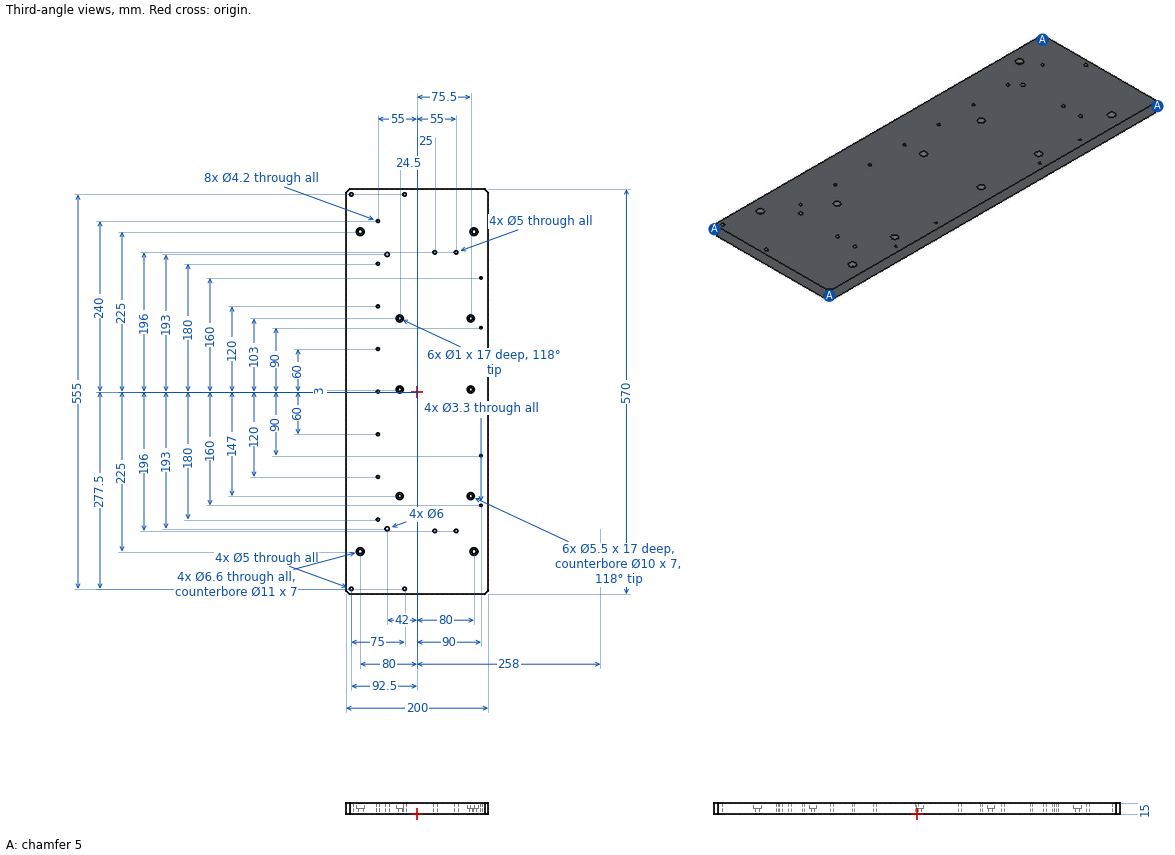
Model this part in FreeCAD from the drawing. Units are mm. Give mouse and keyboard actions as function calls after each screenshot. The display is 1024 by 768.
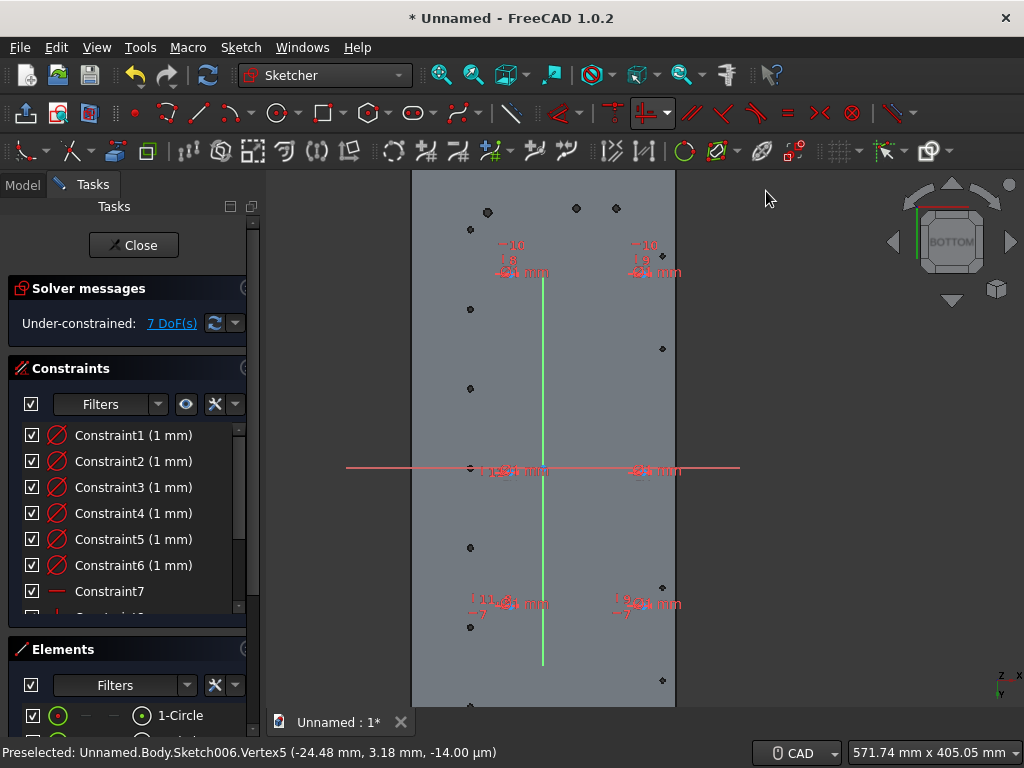
click(643, 606)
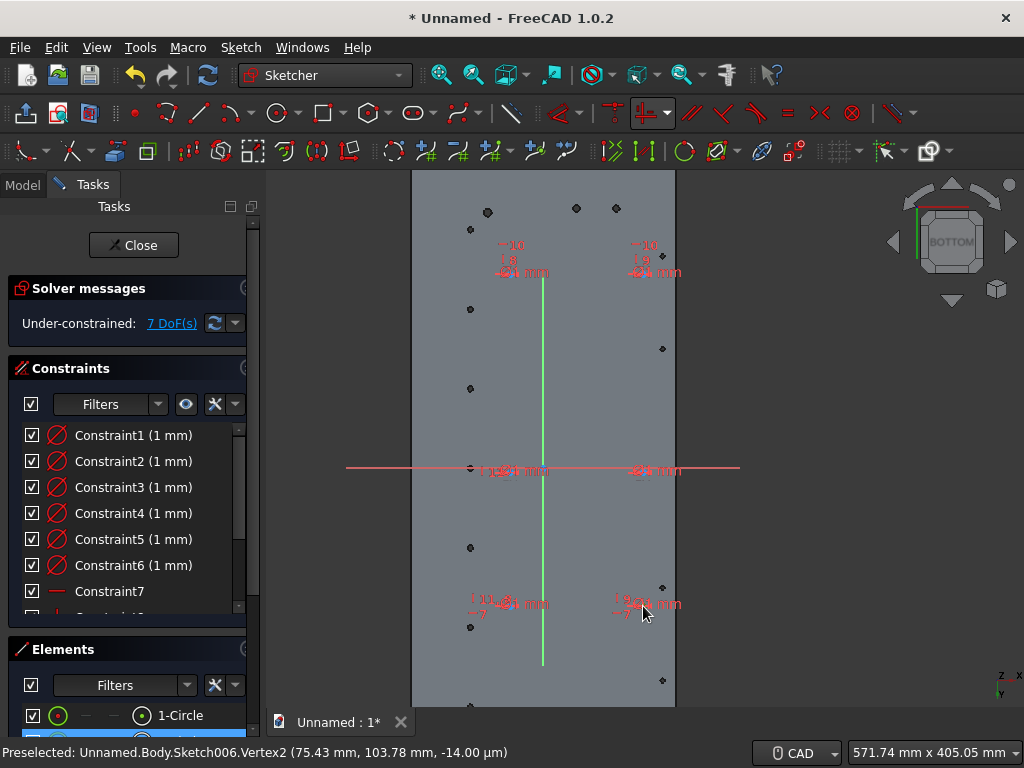
click(643, 473)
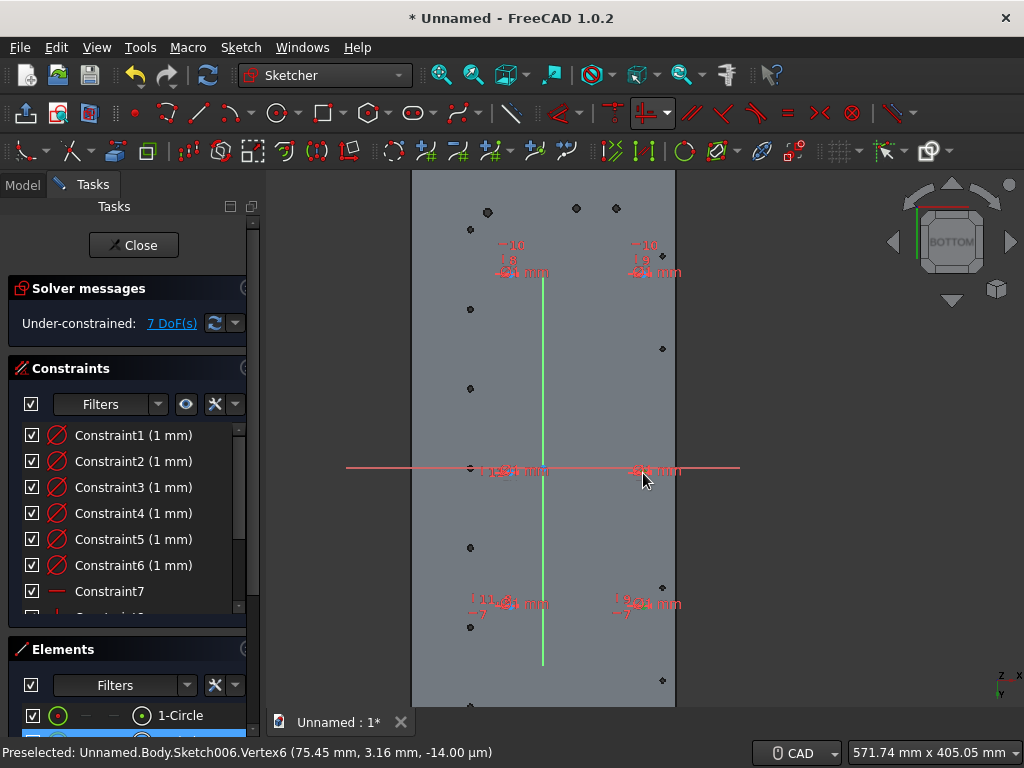
click(670, 114)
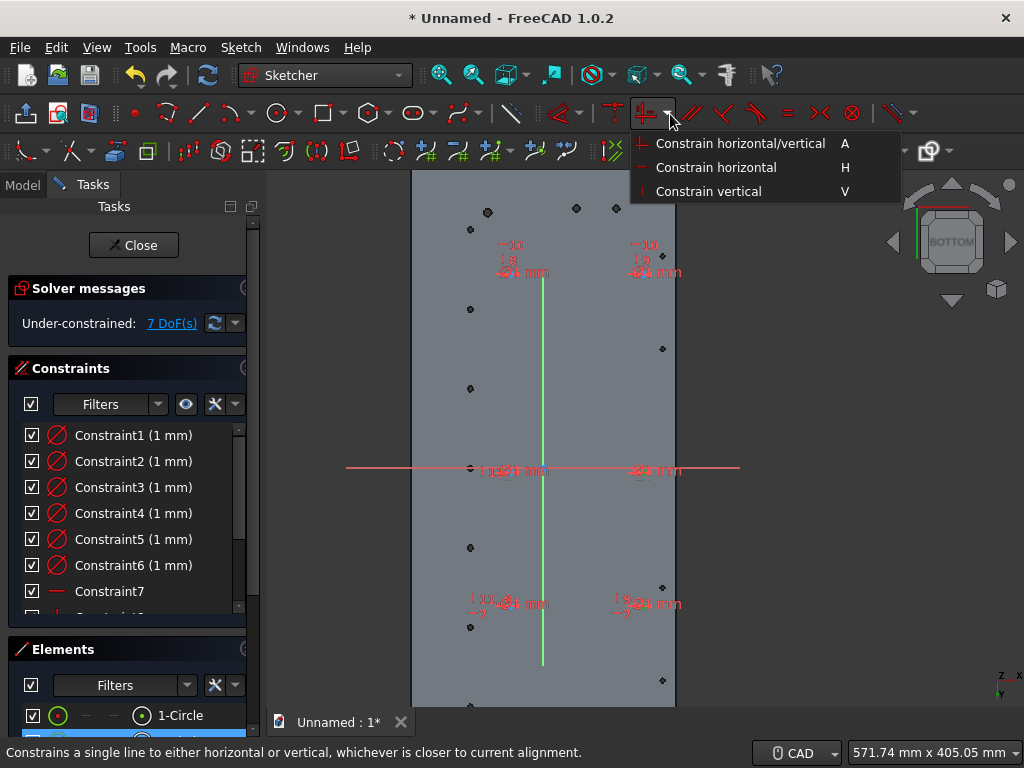
click(766, 191)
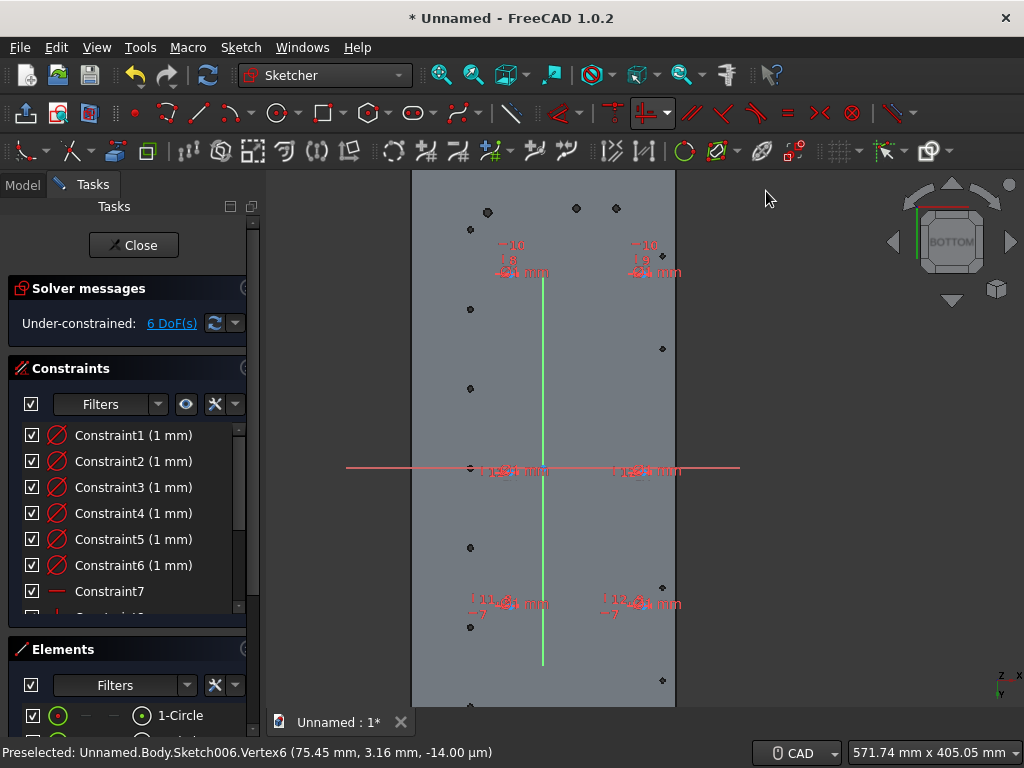
click(511, 473)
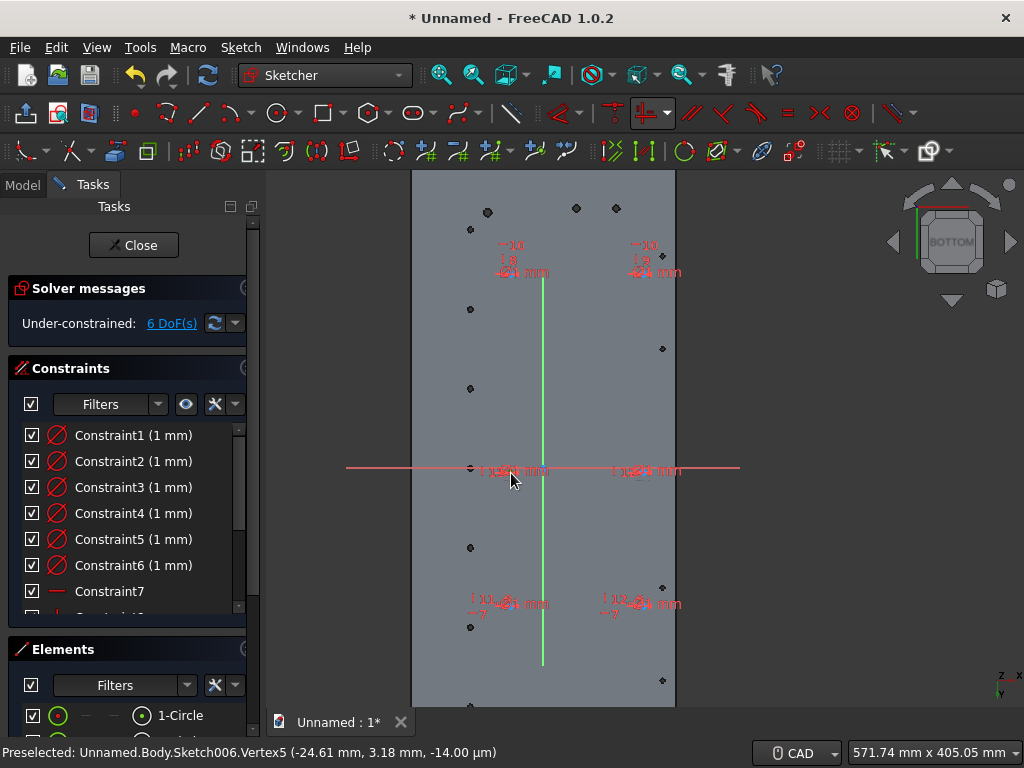
click(643, 473)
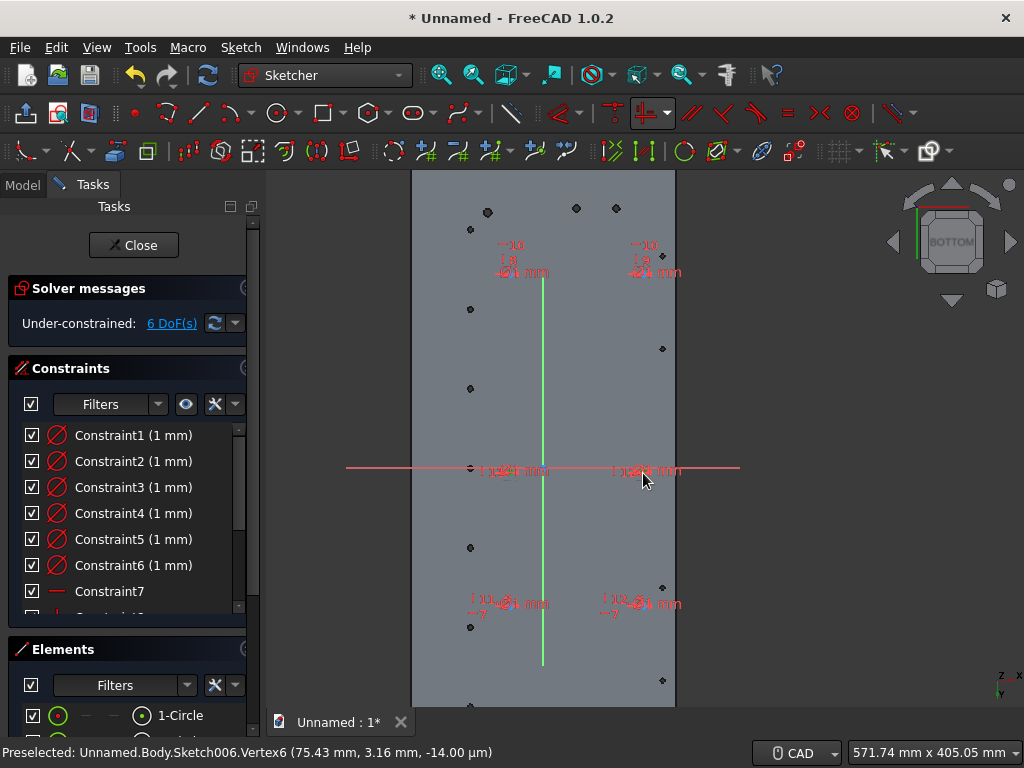
key(h)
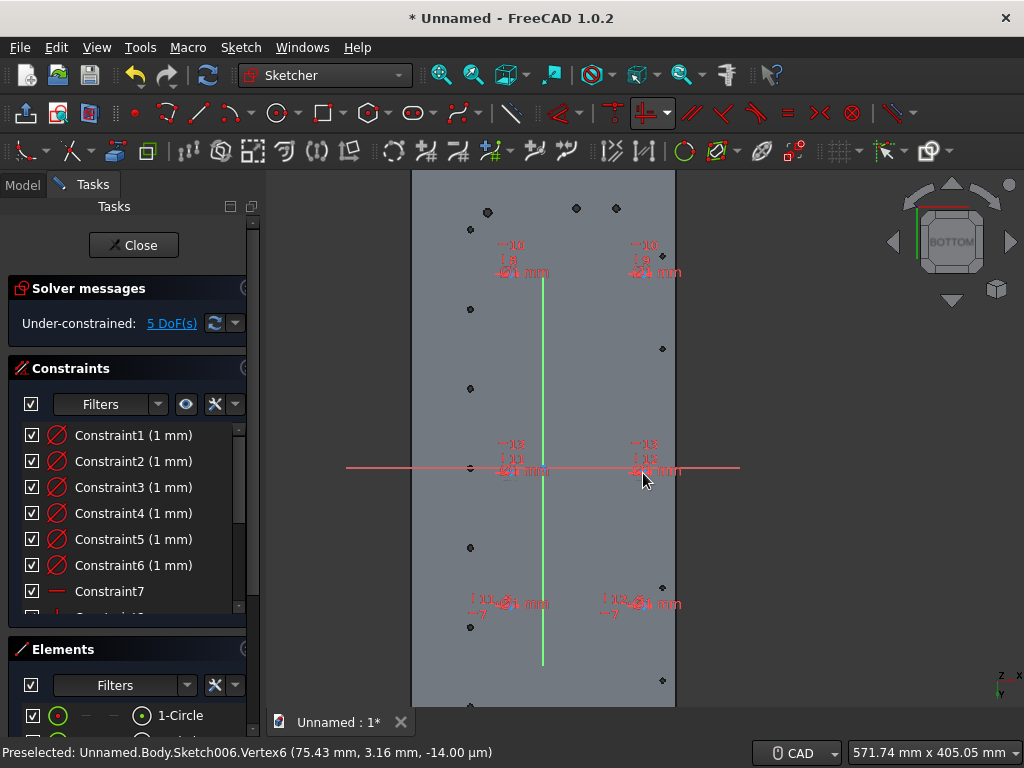
key(d)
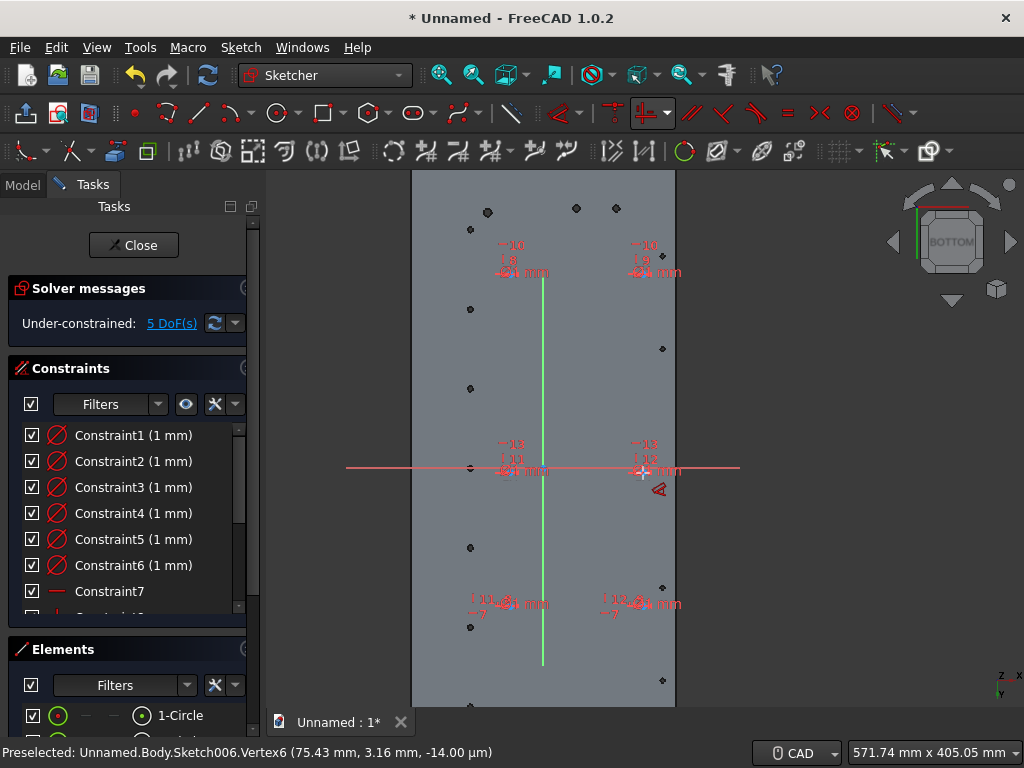
scroll(511, 473, up, 12)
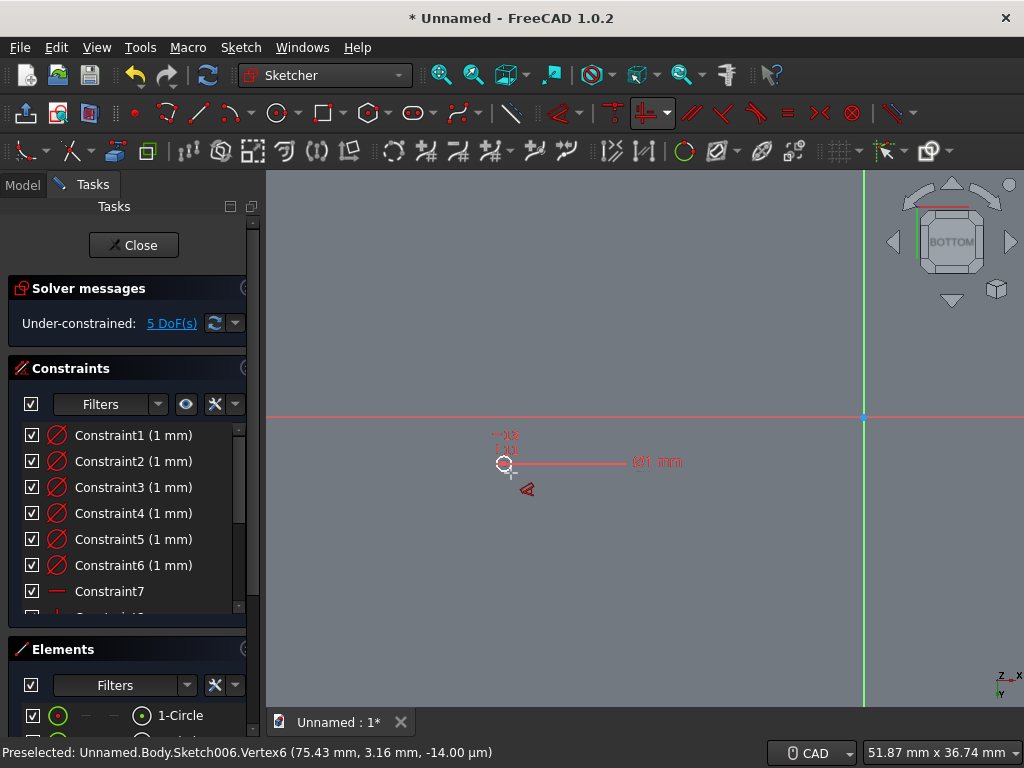
click(504, 464)
click(470, 440)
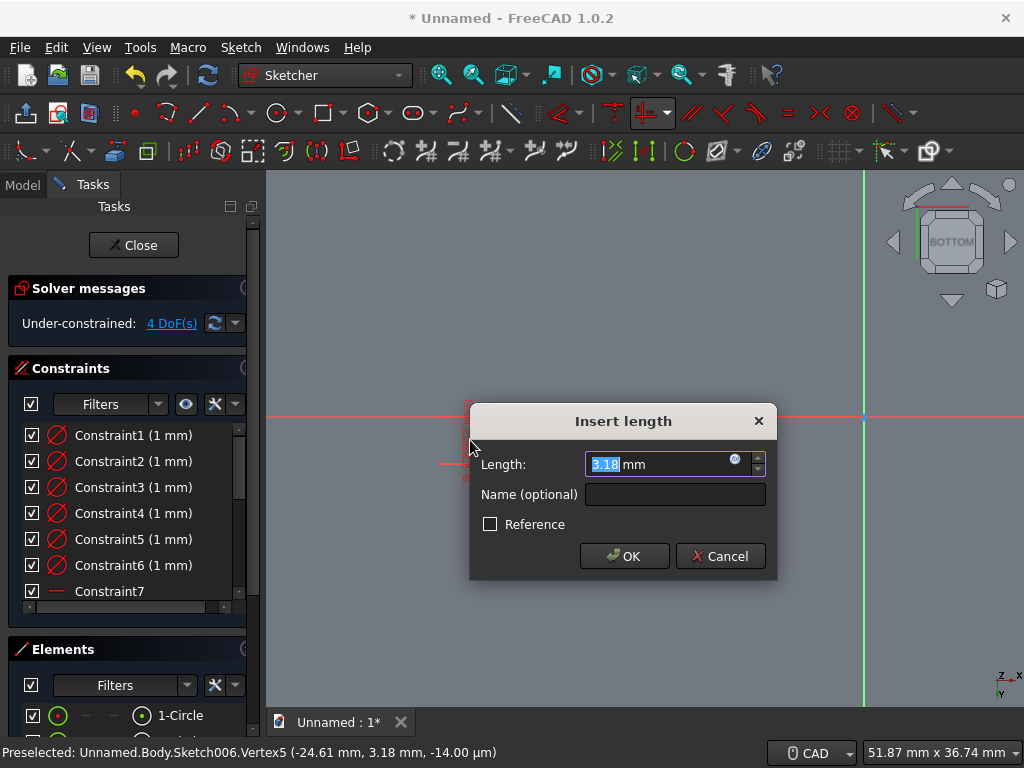
text(3)
key(Return)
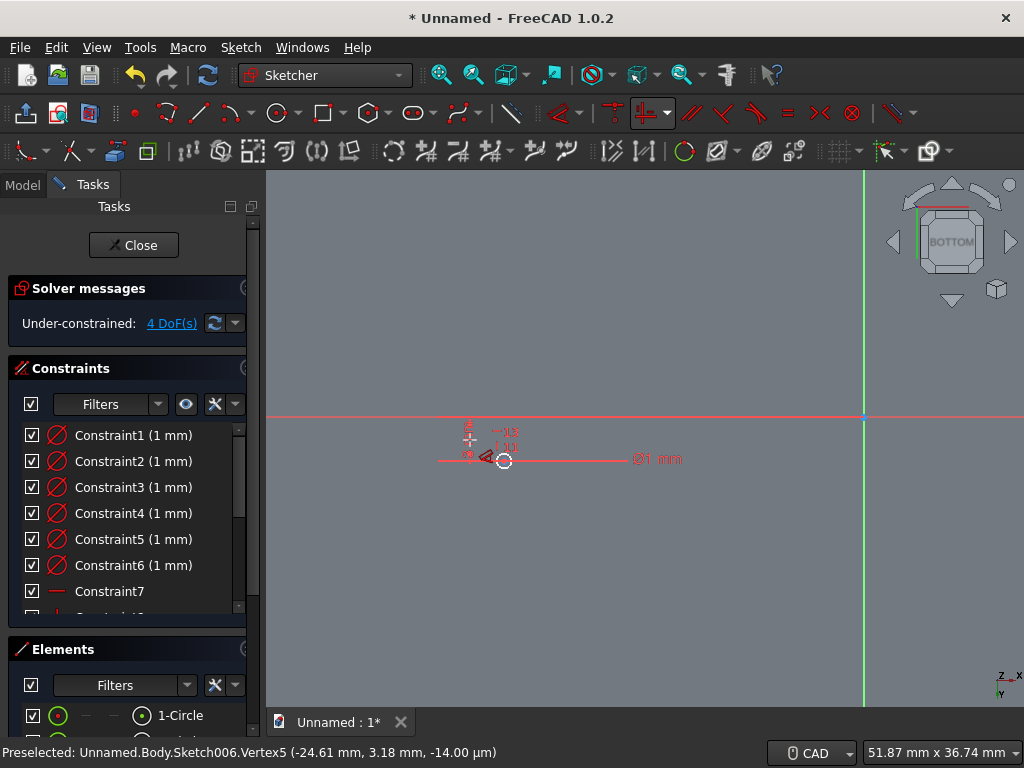
scroll(511, 473, down, 12)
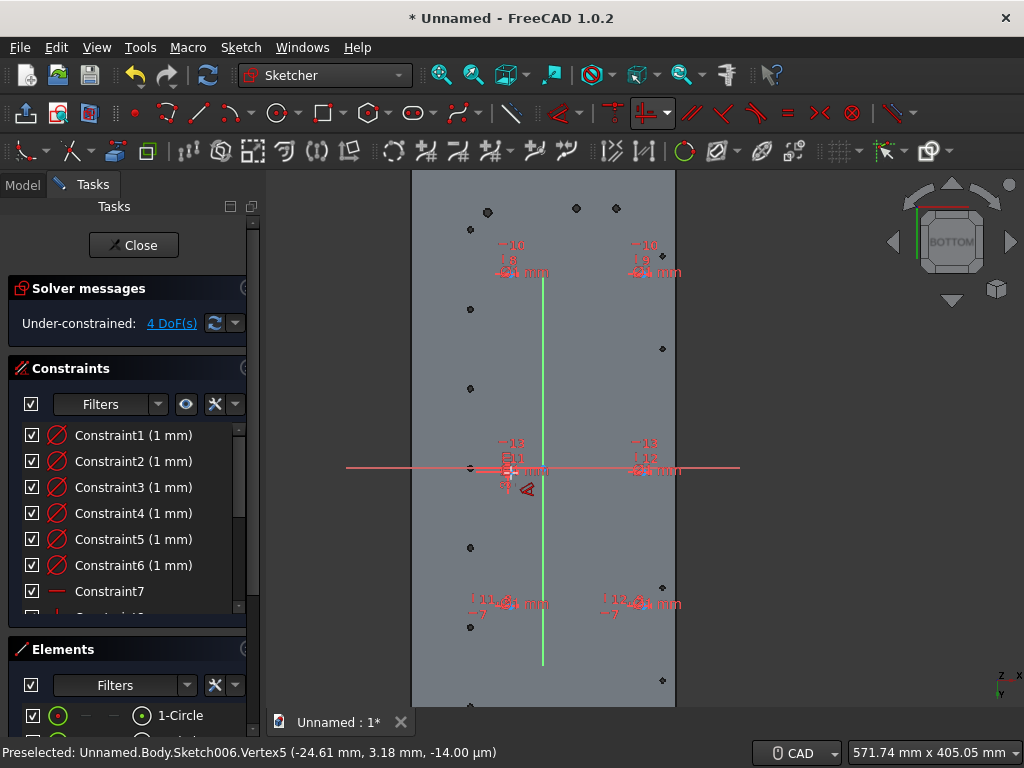
click(511, 606)
click(477, 537)